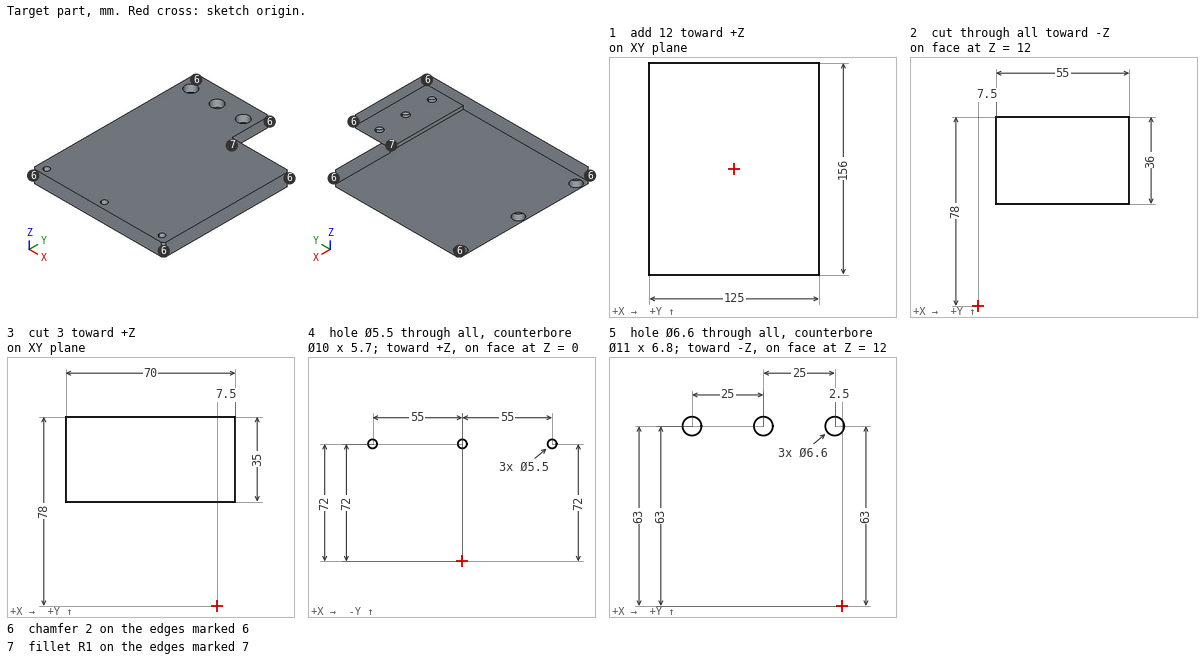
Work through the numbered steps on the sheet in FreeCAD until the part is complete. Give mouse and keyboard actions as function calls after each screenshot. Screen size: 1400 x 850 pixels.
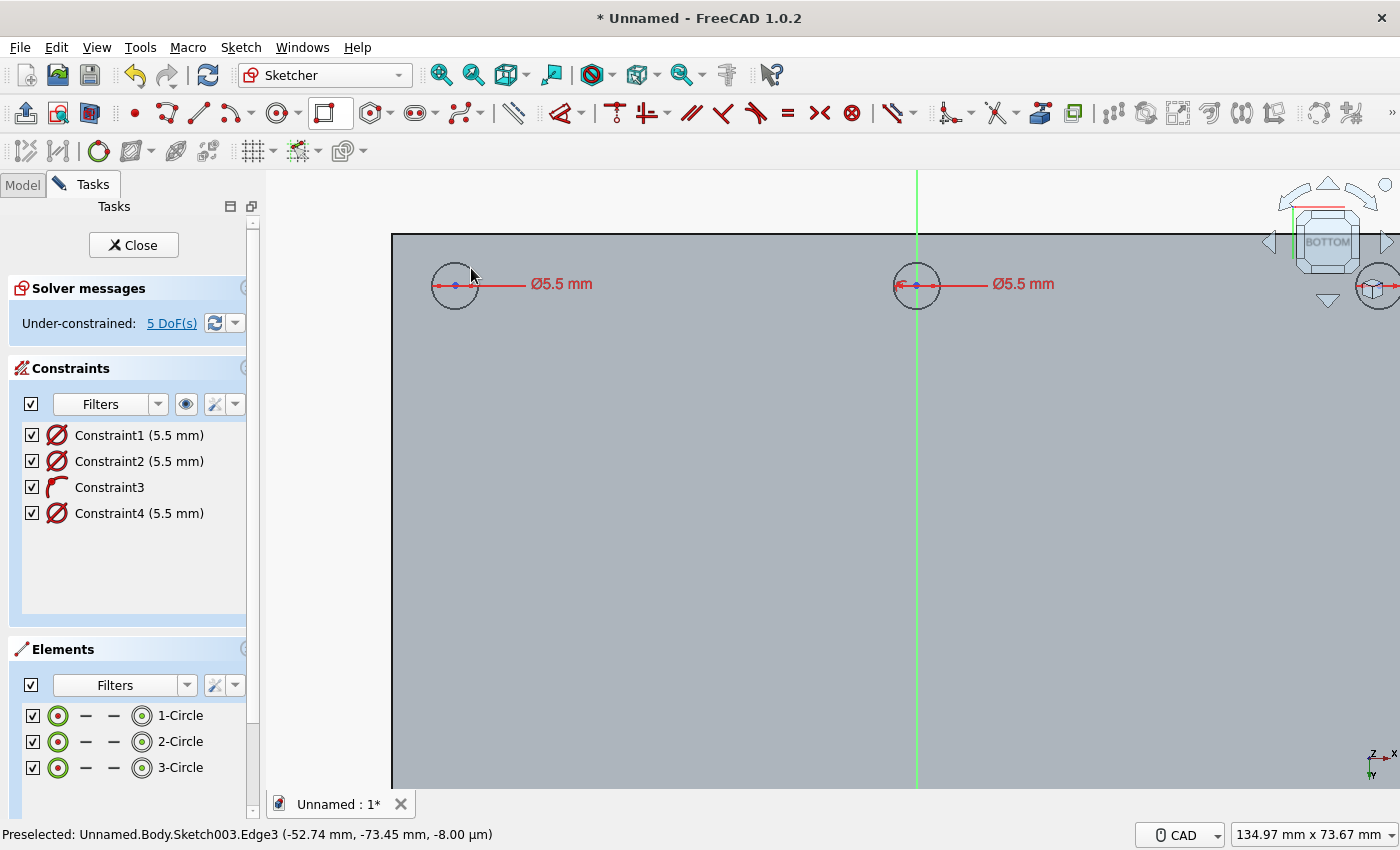
click(560, 114)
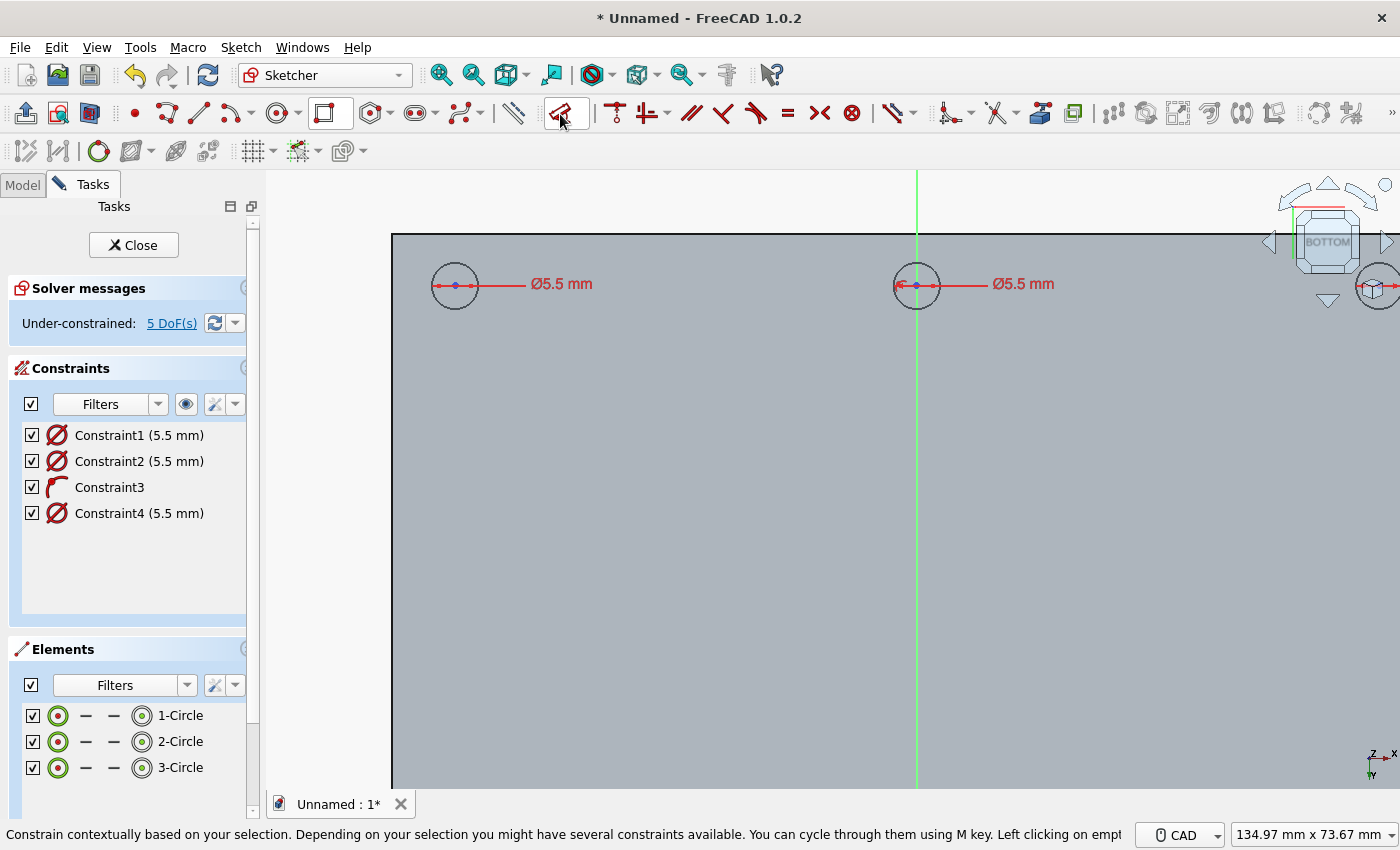
scroll(455, 284, down, 2)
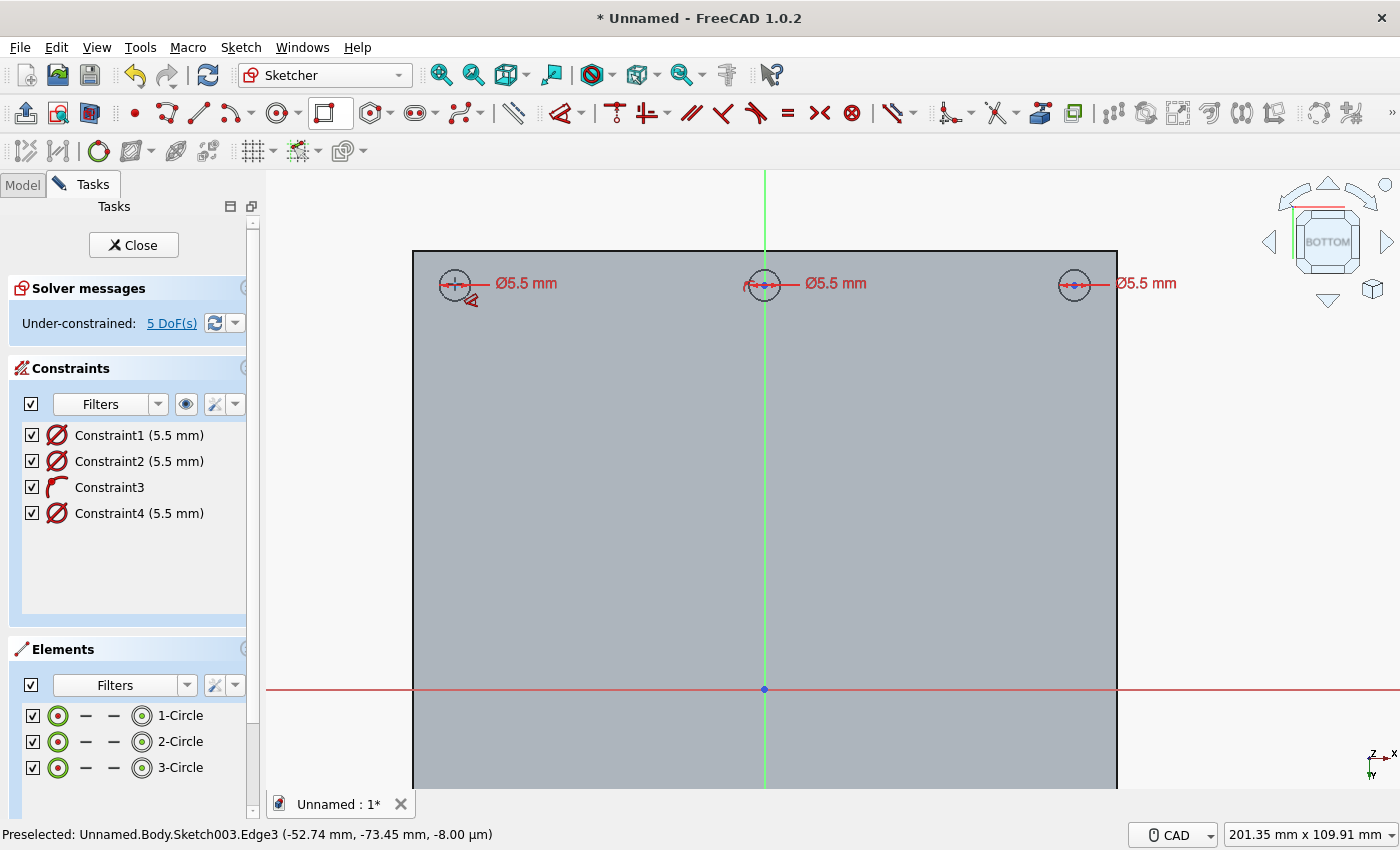
click(1075, 285)
click(920, 724)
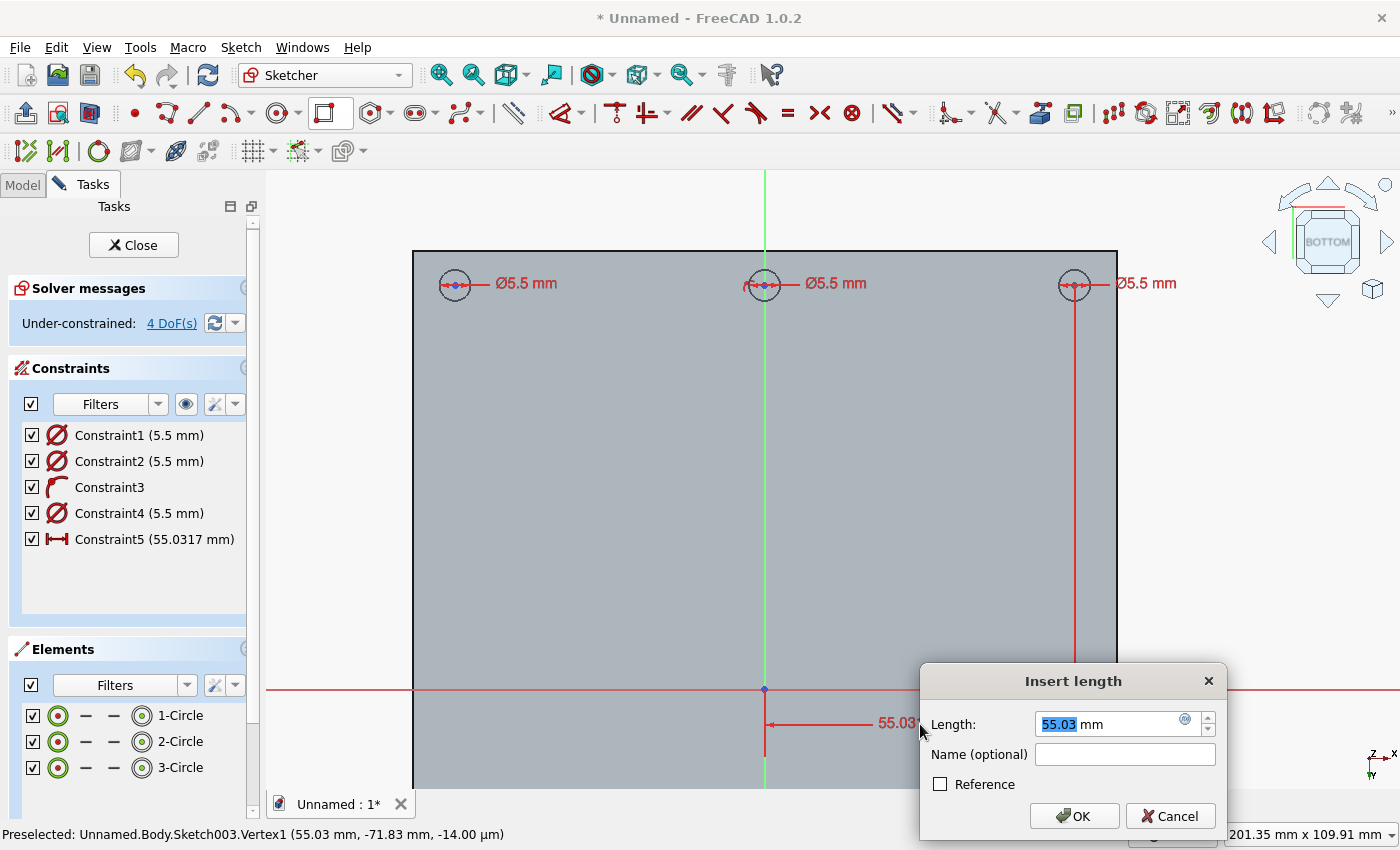
text(55)
key(Return)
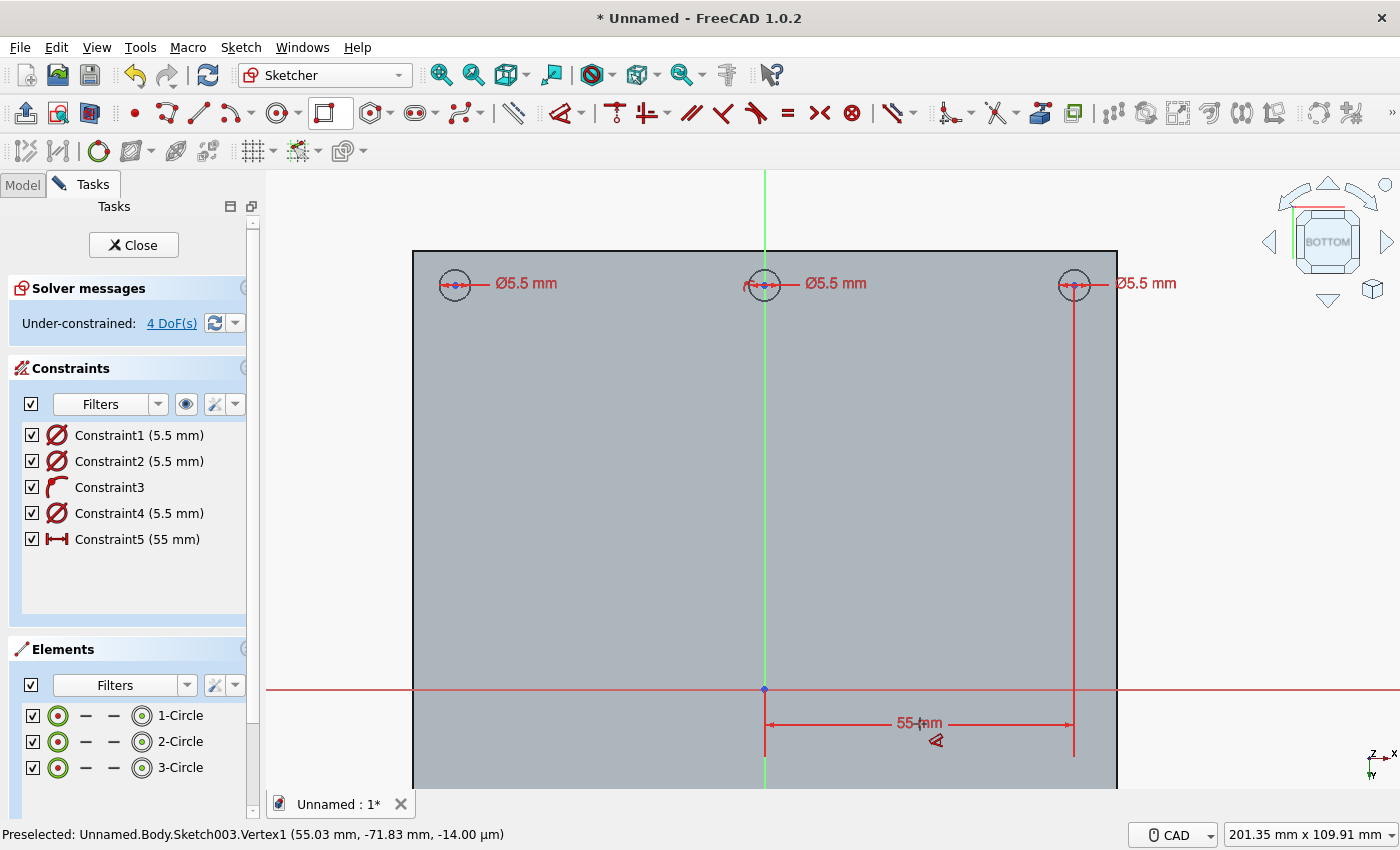
click(1074, 285)
click(1108, 488)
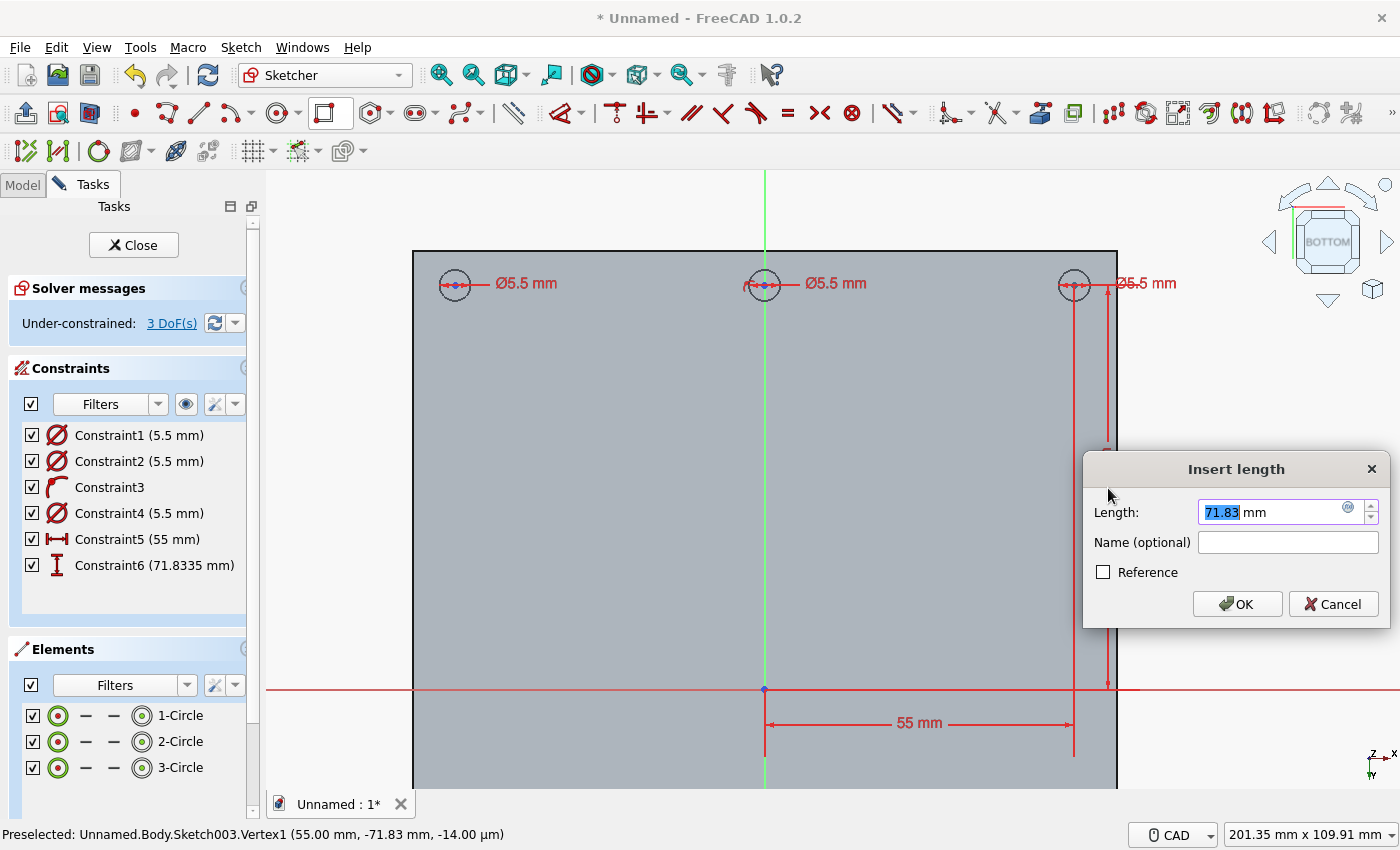
text(72)
key(Return)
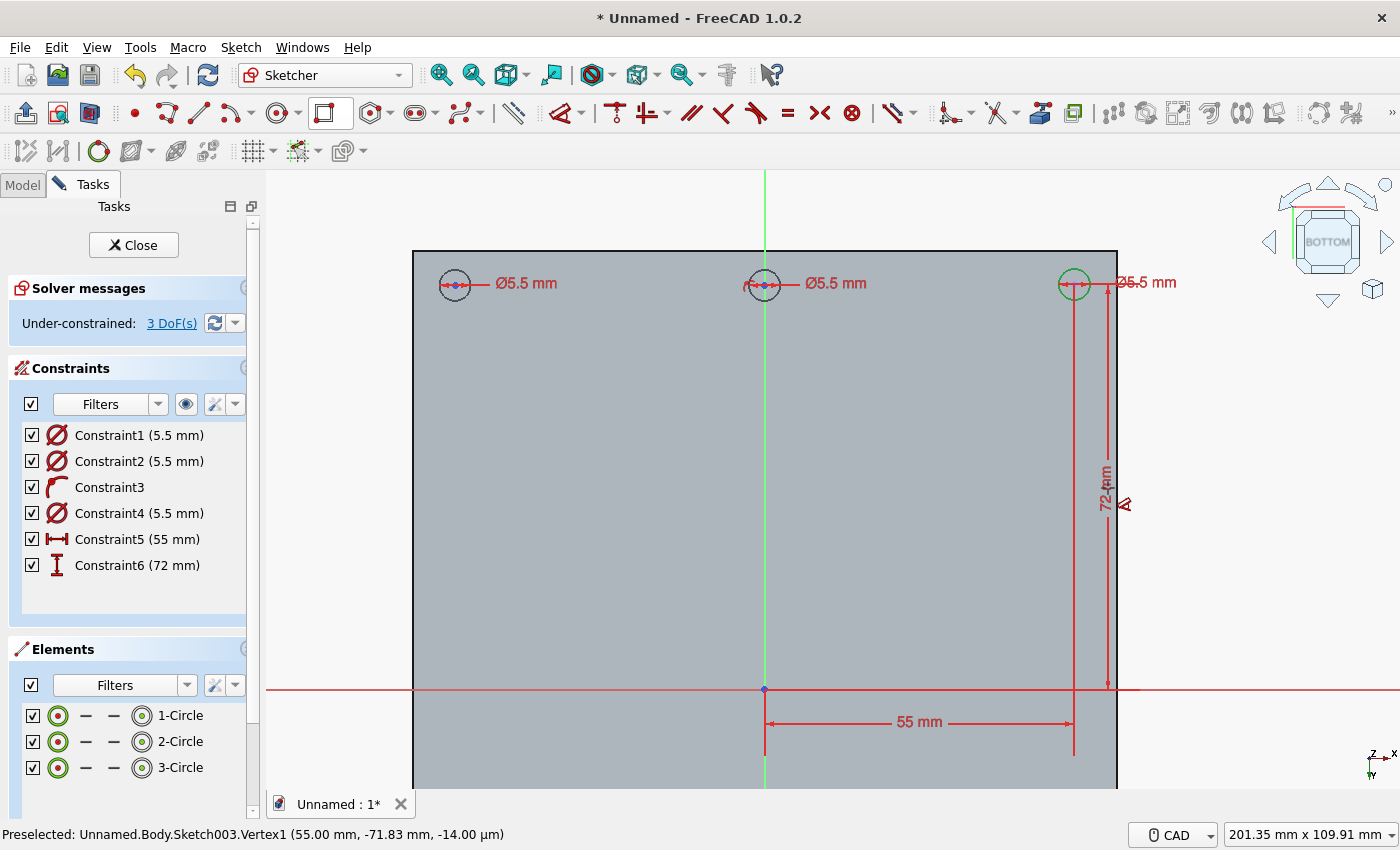
click(765, 285)
click(799, 488)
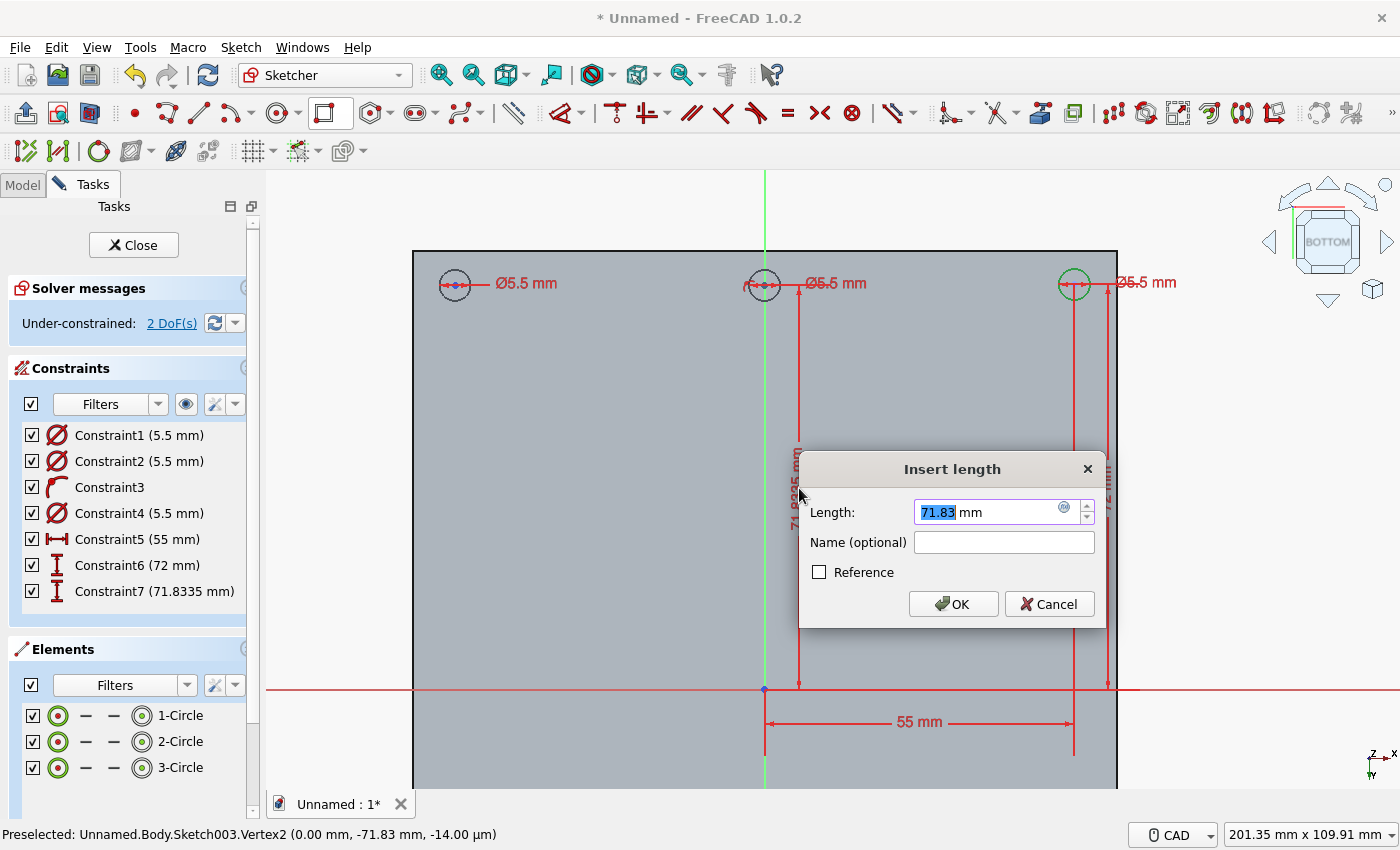
text(72)
key(Return)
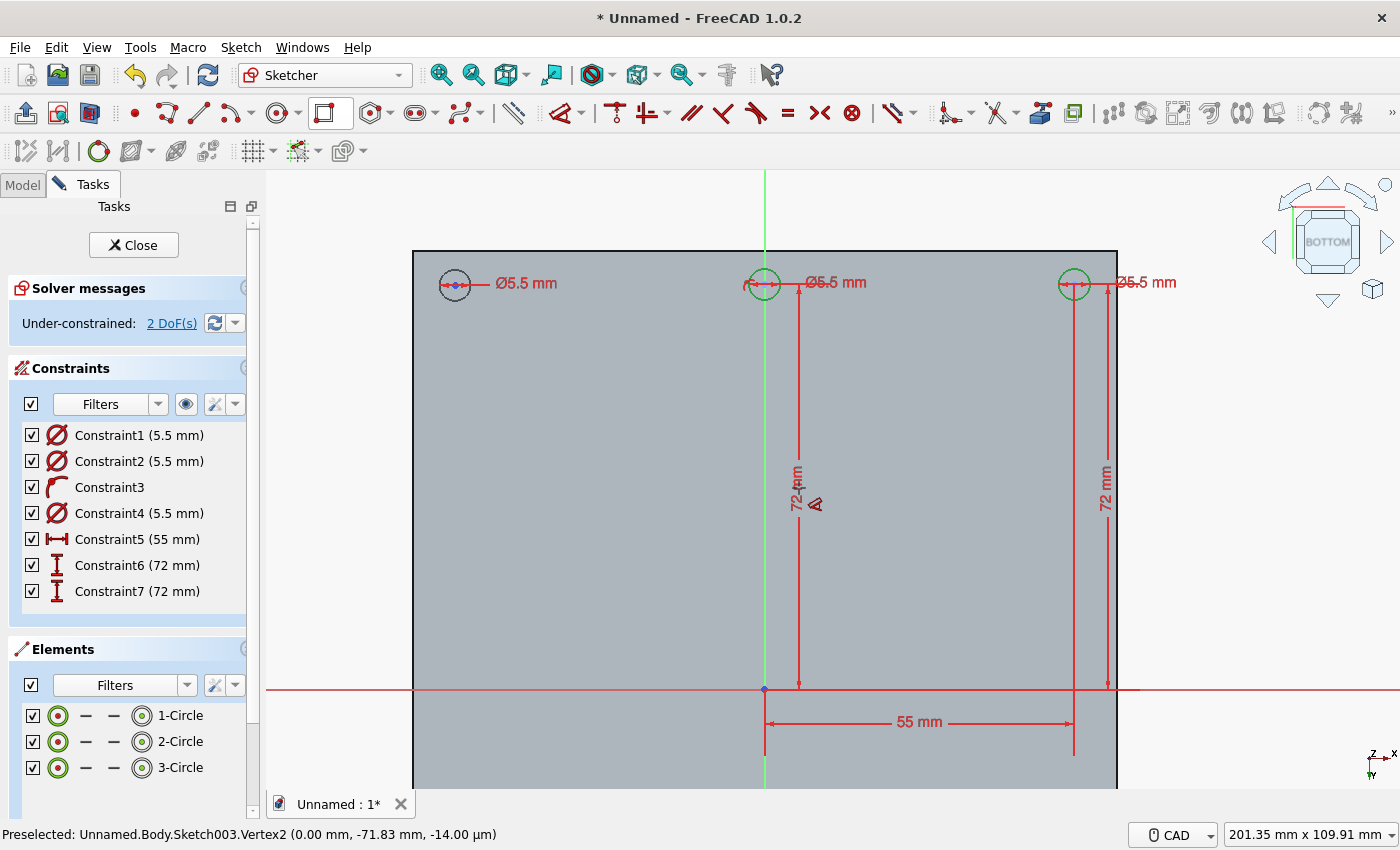
click(455, 285)
click(610, 724)